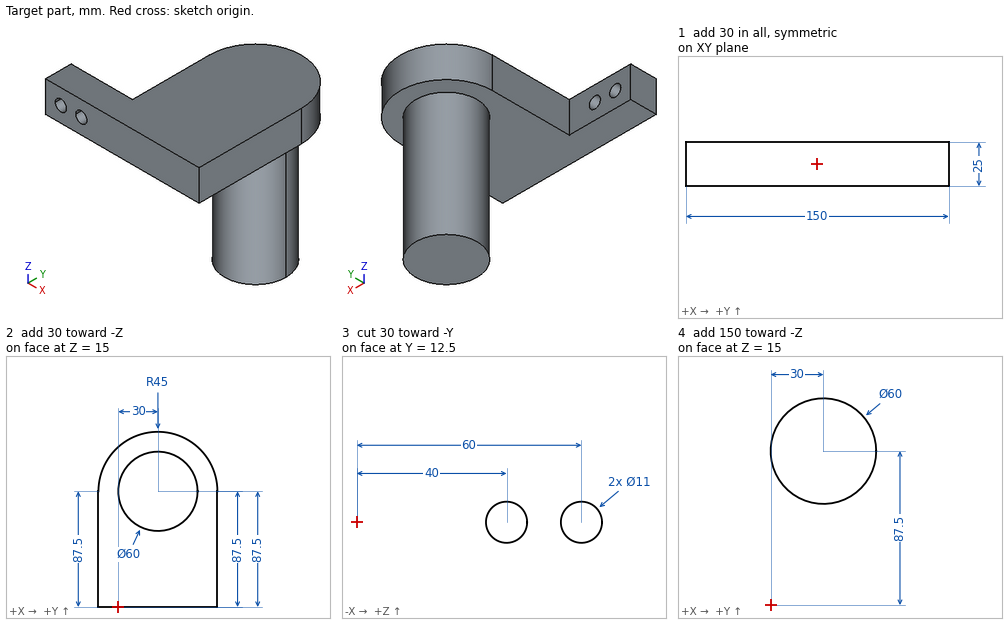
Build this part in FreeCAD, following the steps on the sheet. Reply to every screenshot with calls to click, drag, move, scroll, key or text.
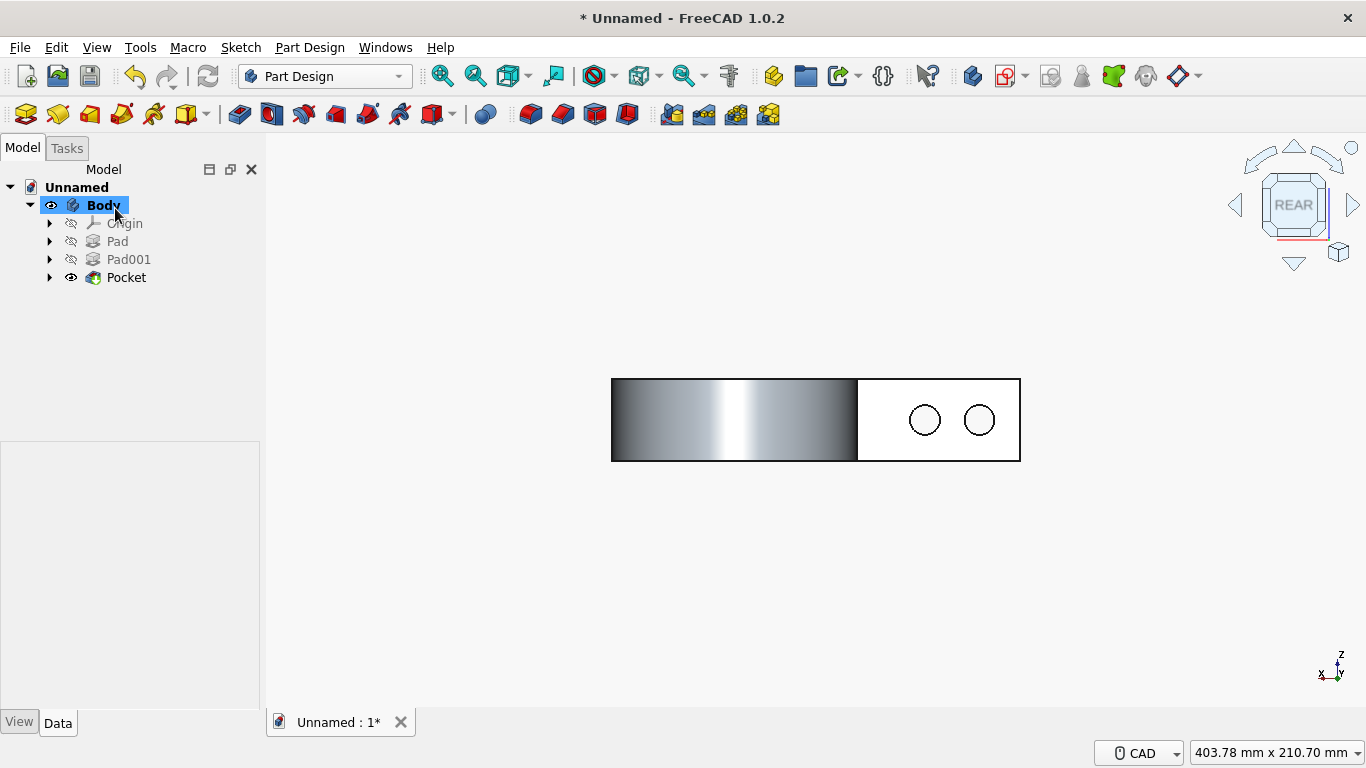
click(444, 76)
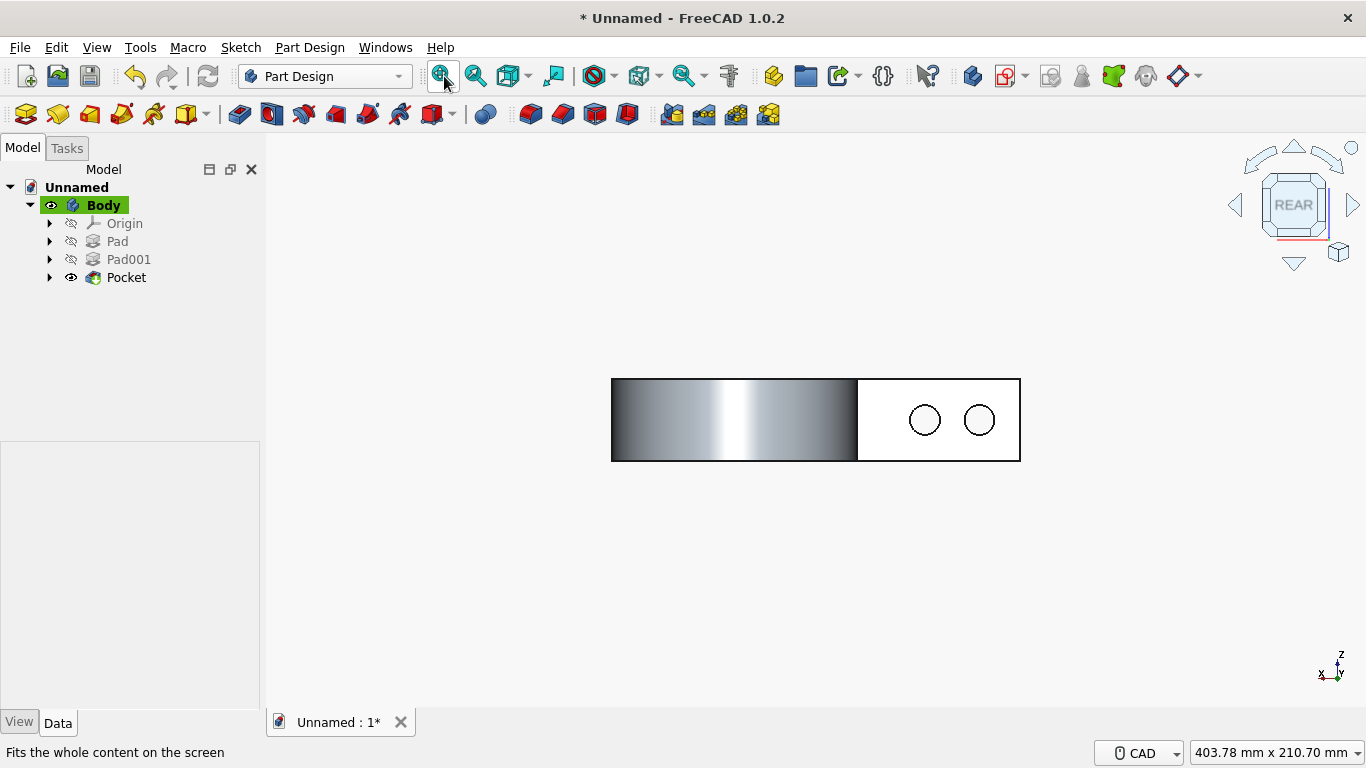
key(0)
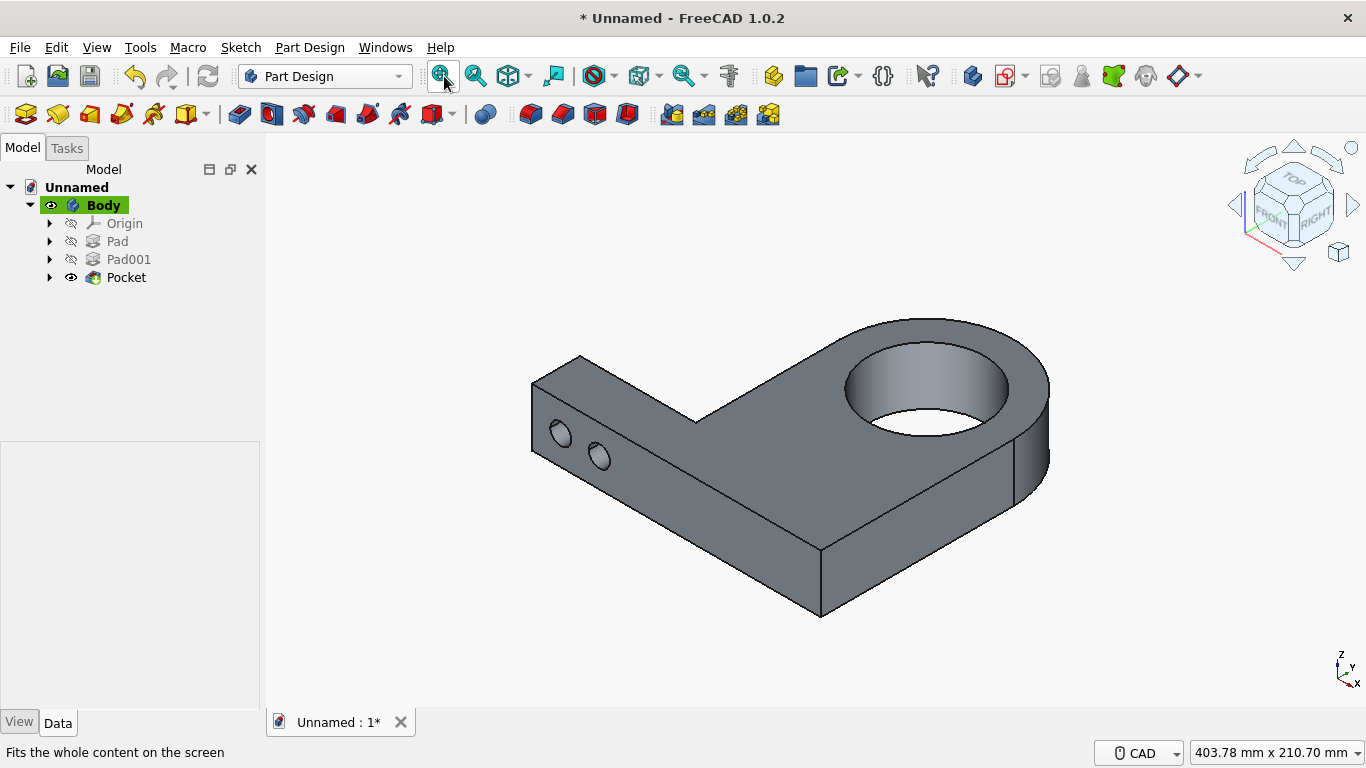
click(819, 479)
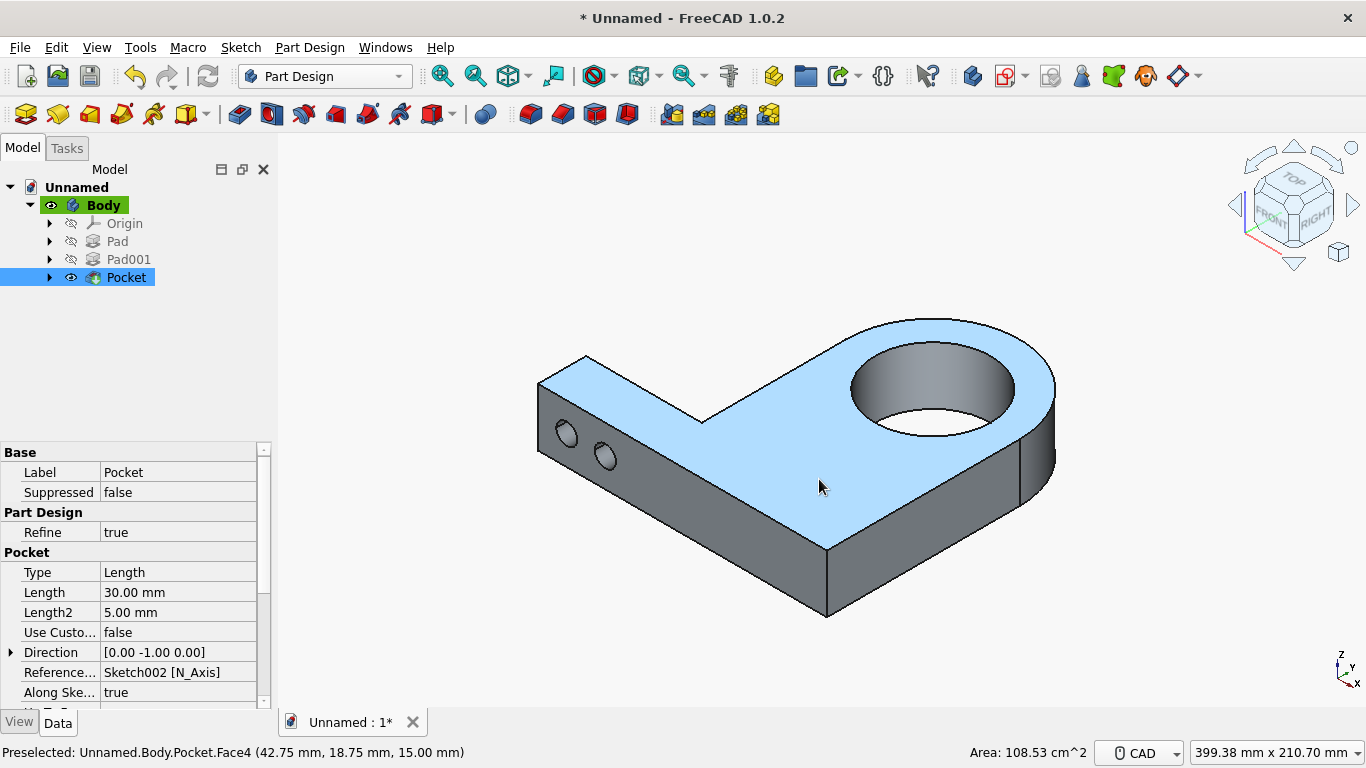
click(1006, 76)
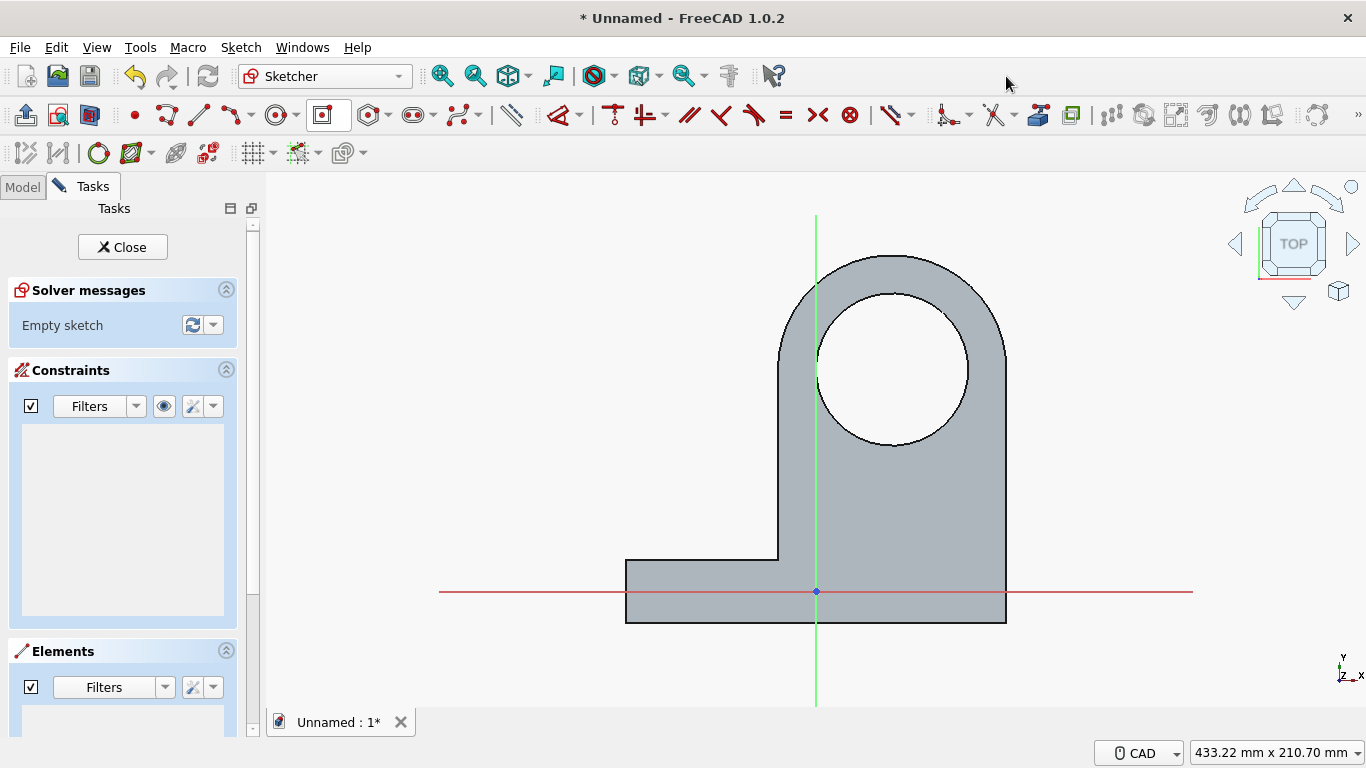
click(276, 116)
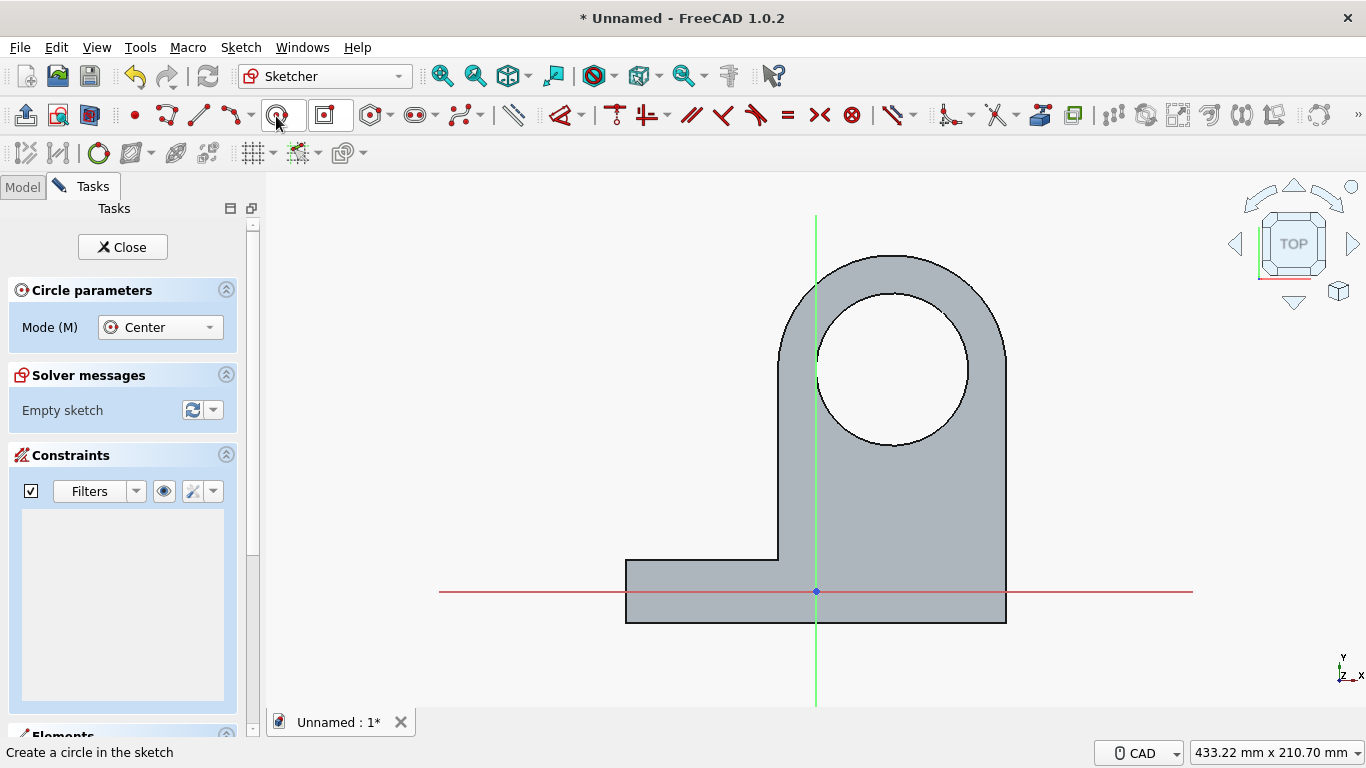
click(892, 370)
click(946, 316)
key(Escape)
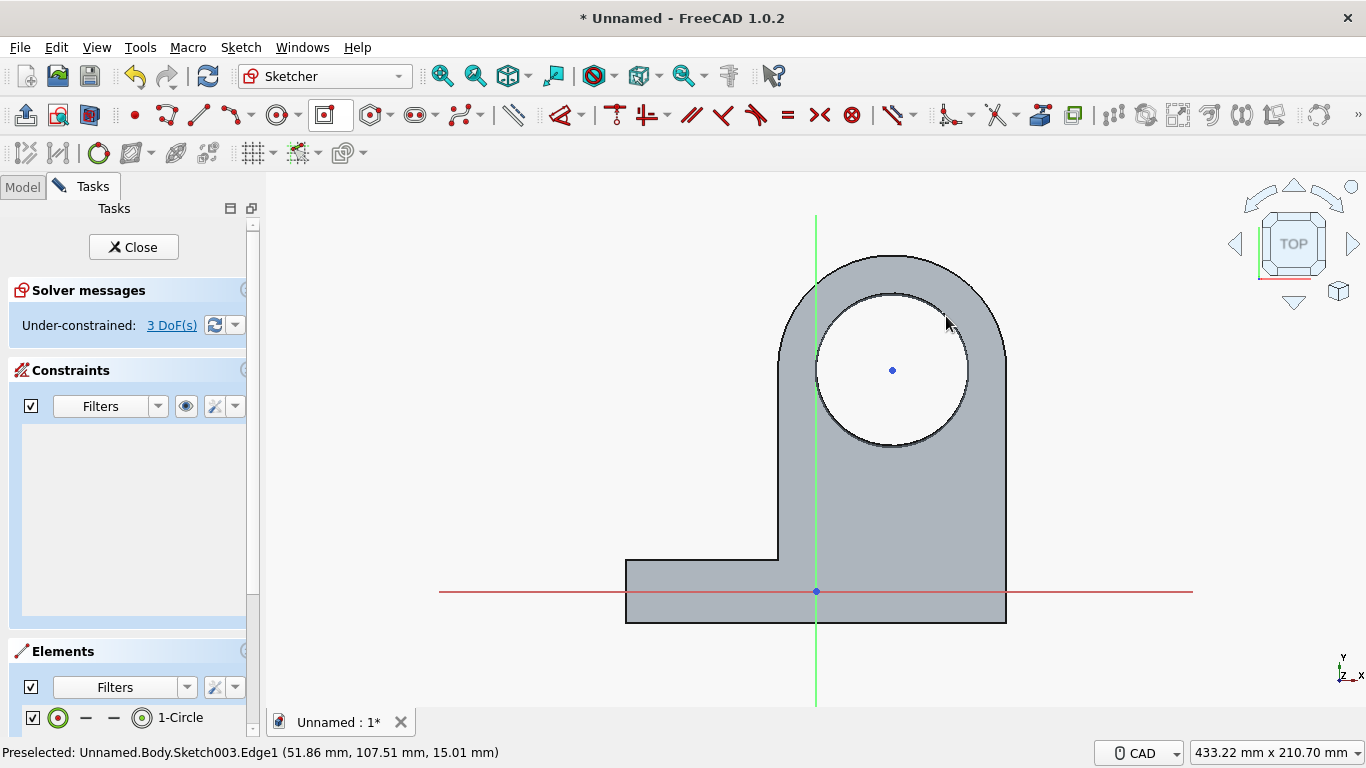
key(d)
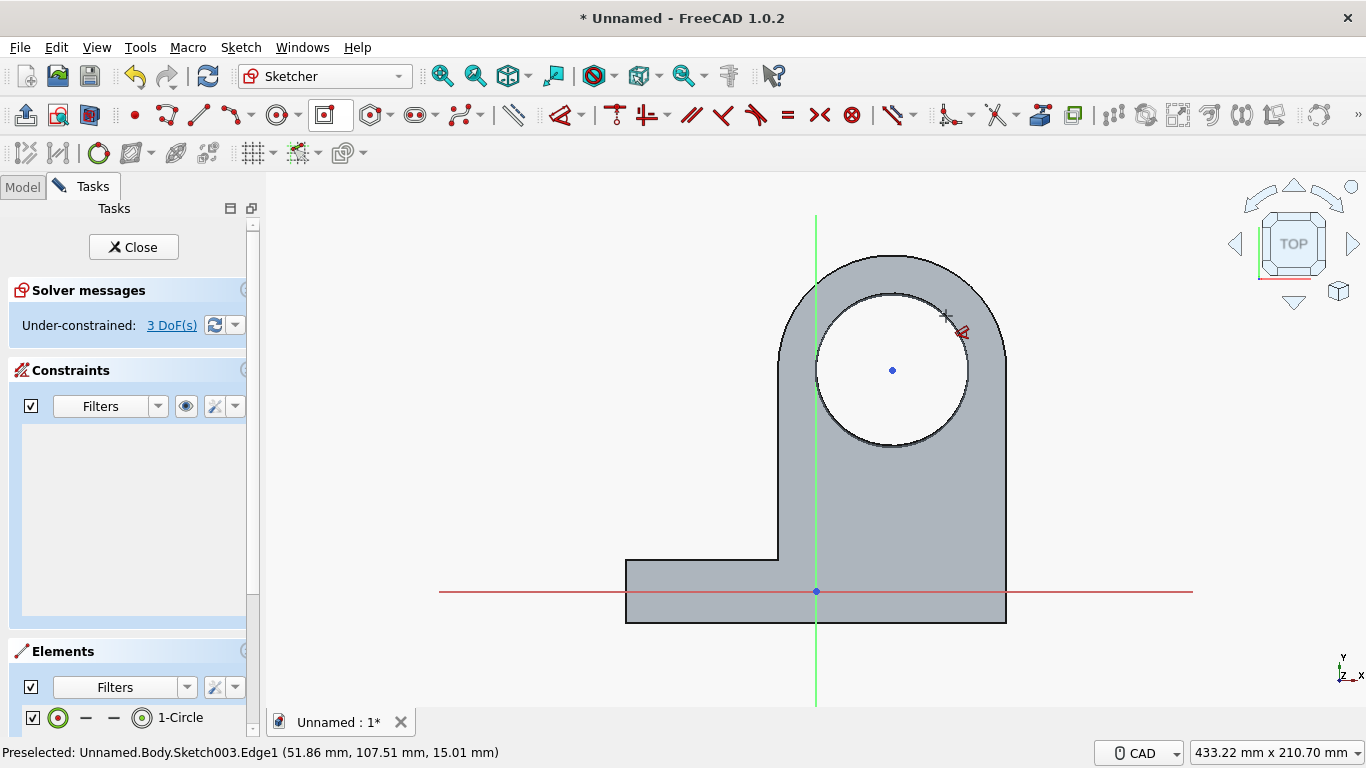
click(946, 317)
click(969, 294)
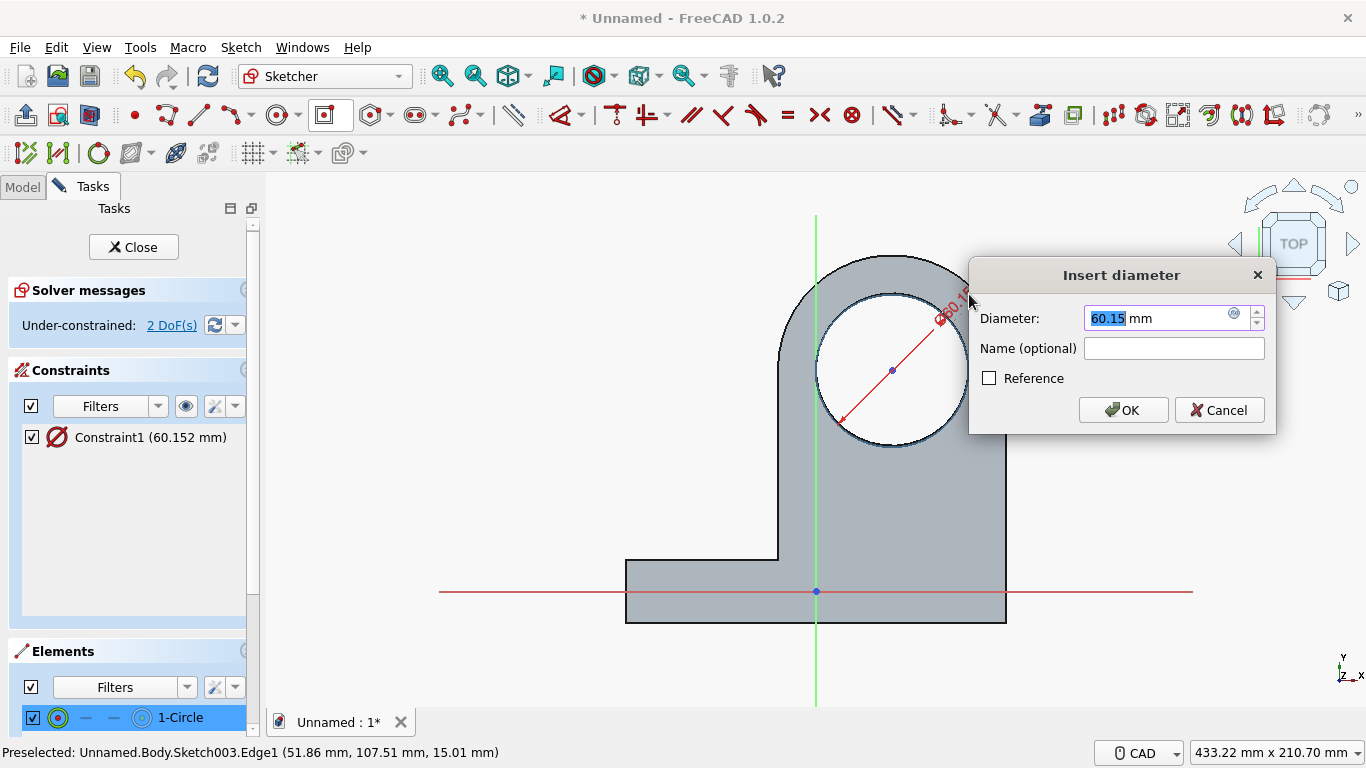
text(60)
key(Return)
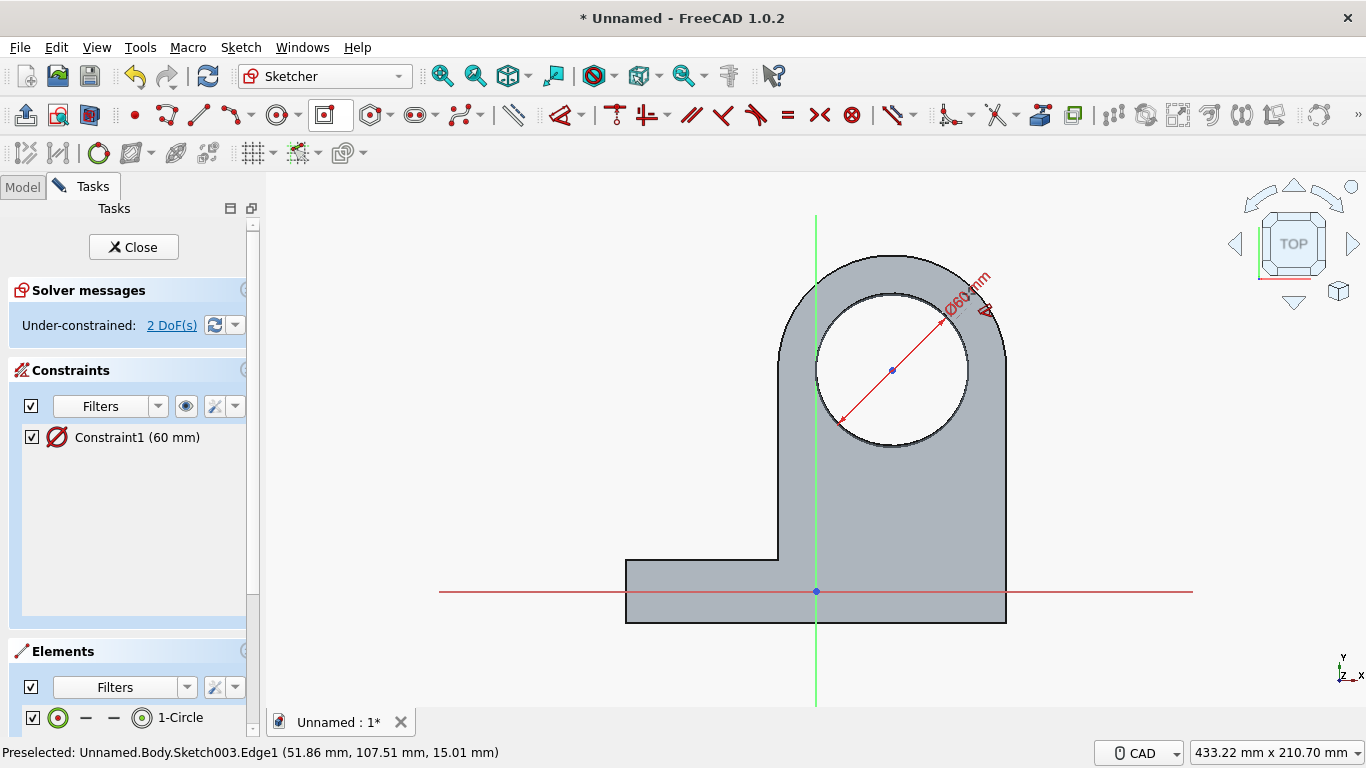
click(892, 371)
click(854, 626)